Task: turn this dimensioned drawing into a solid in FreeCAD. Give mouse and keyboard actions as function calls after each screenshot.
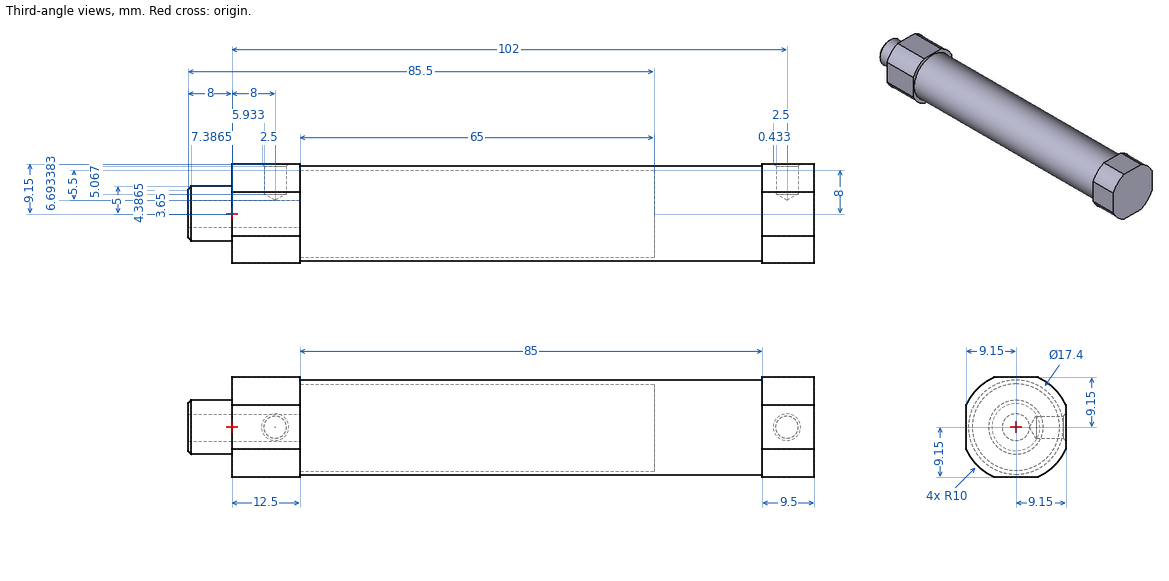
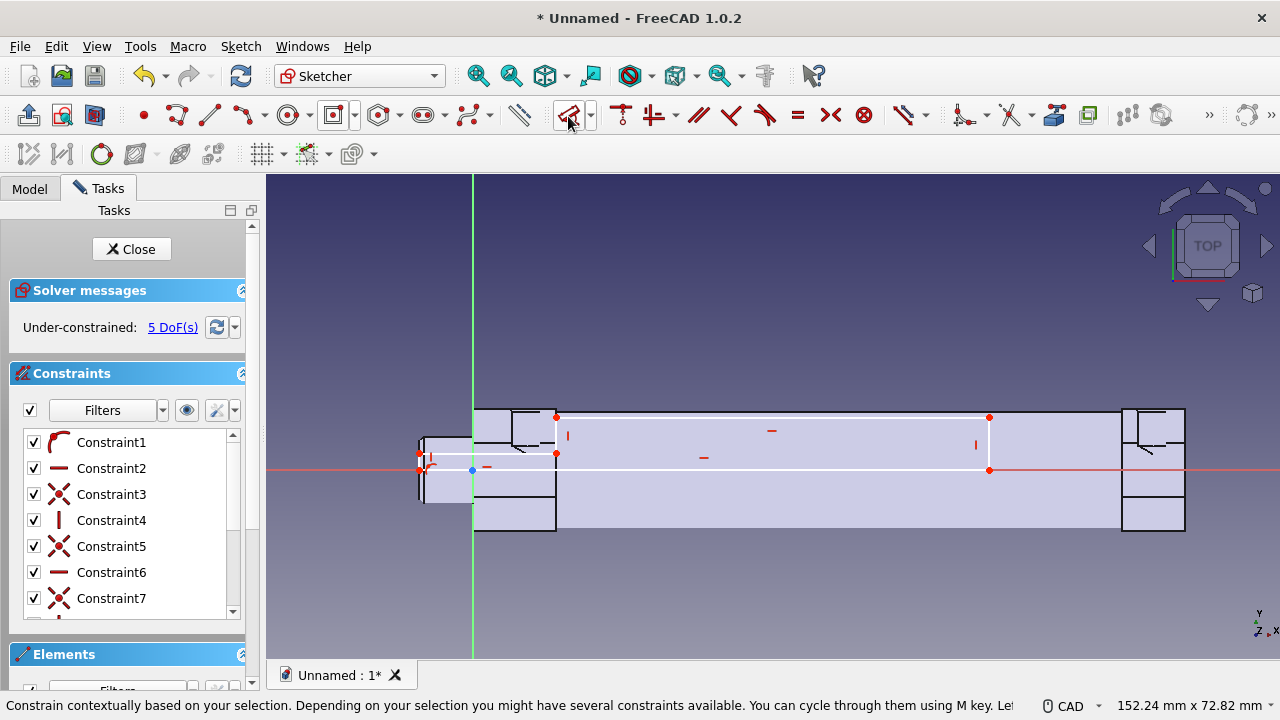
click(989, 454)
click(1023, 444)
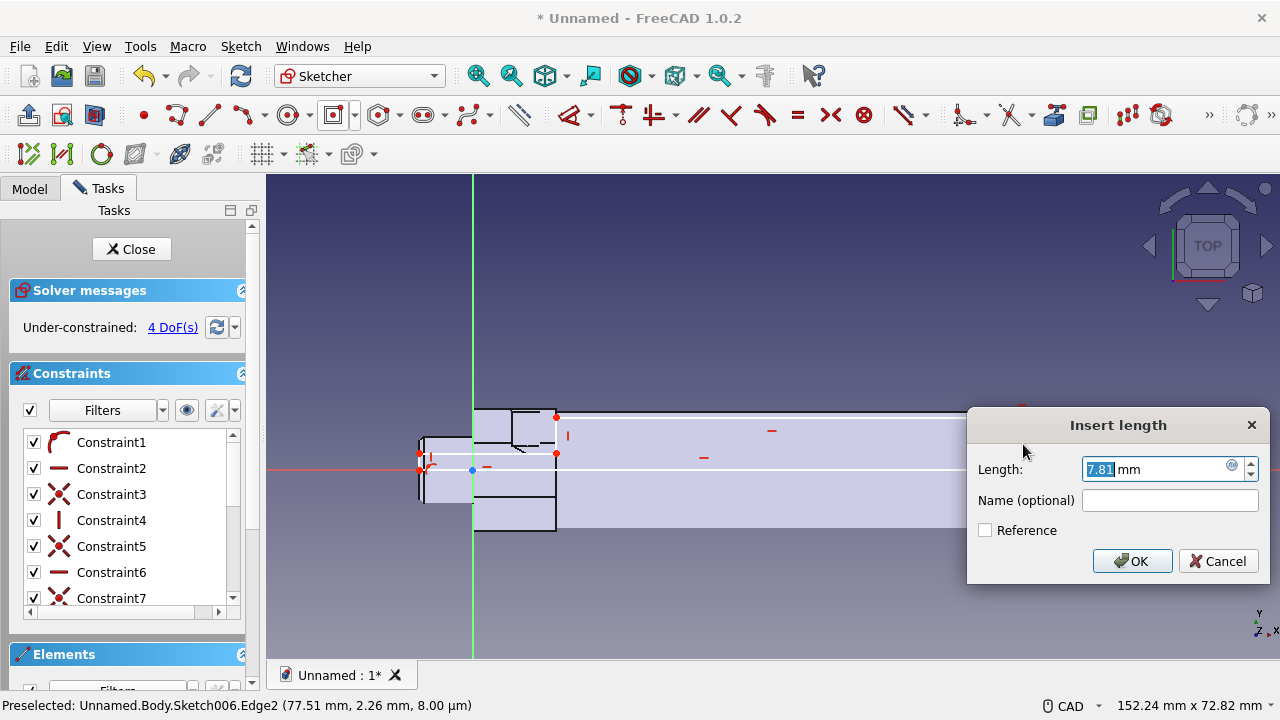
text(8)
key(Return)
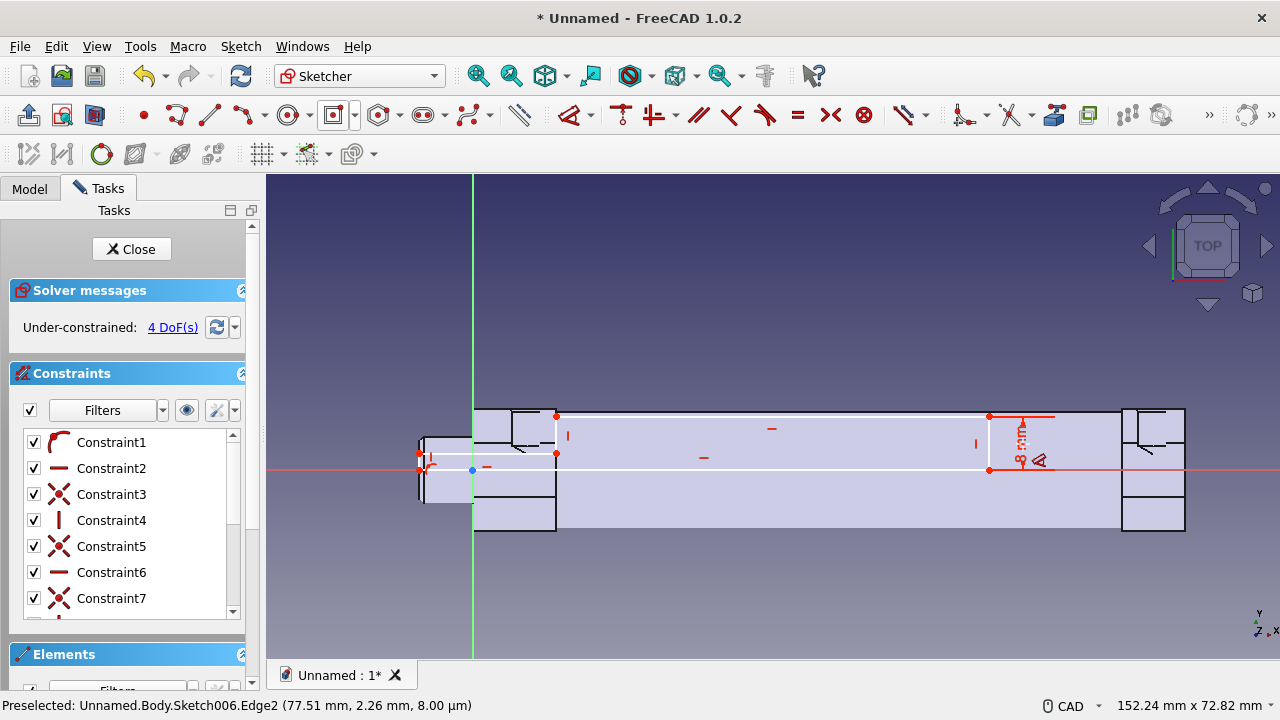
click(859, 417)
click(772, 383)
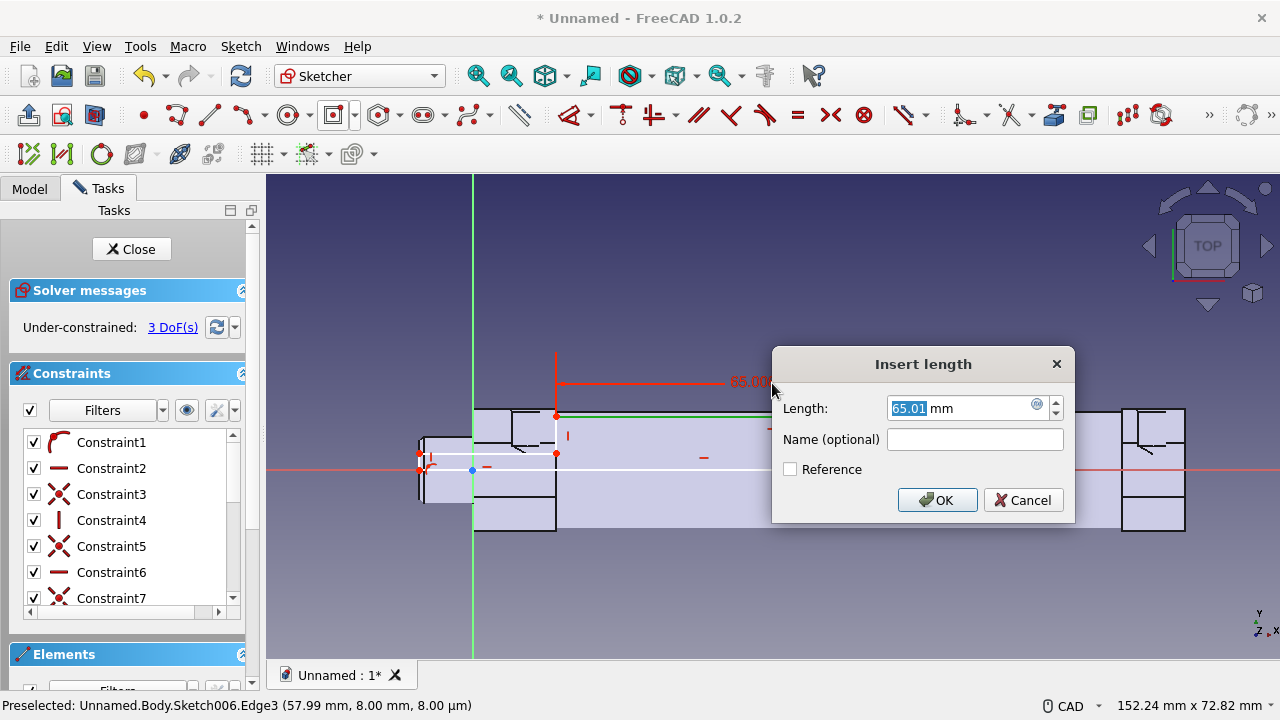
text(65)
key(Return)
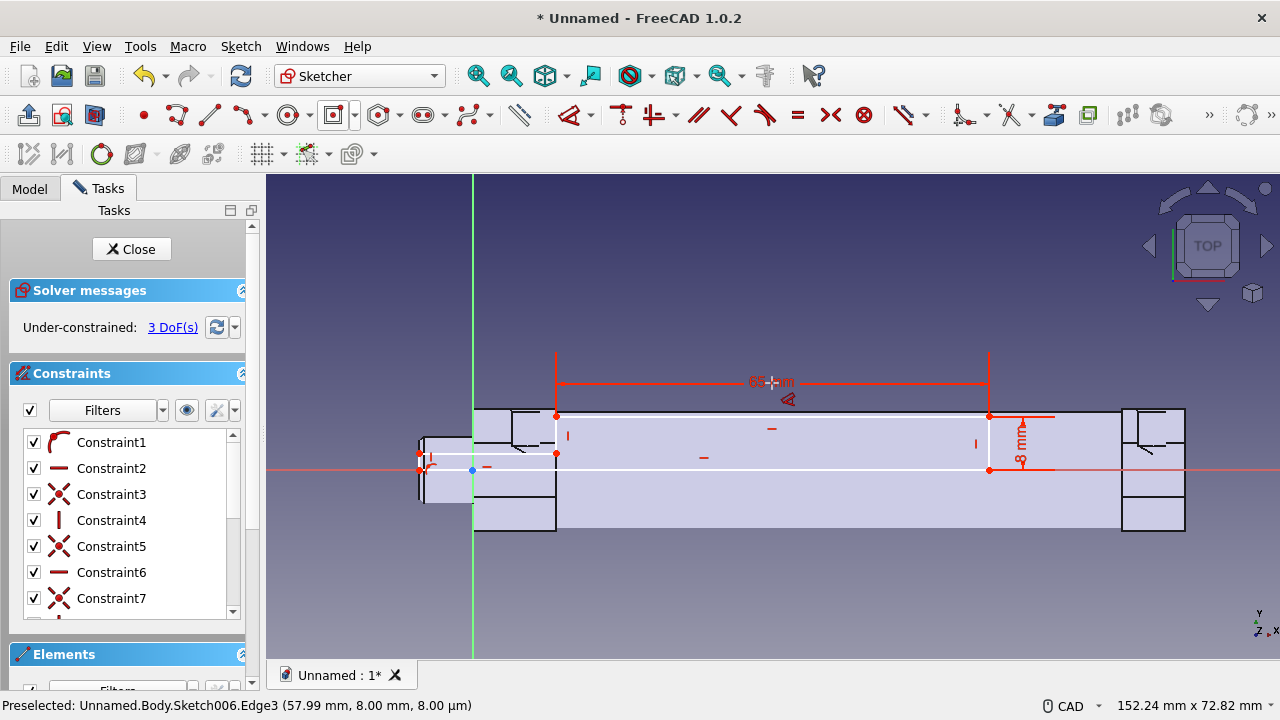
click(419, 470)
click(446, 504)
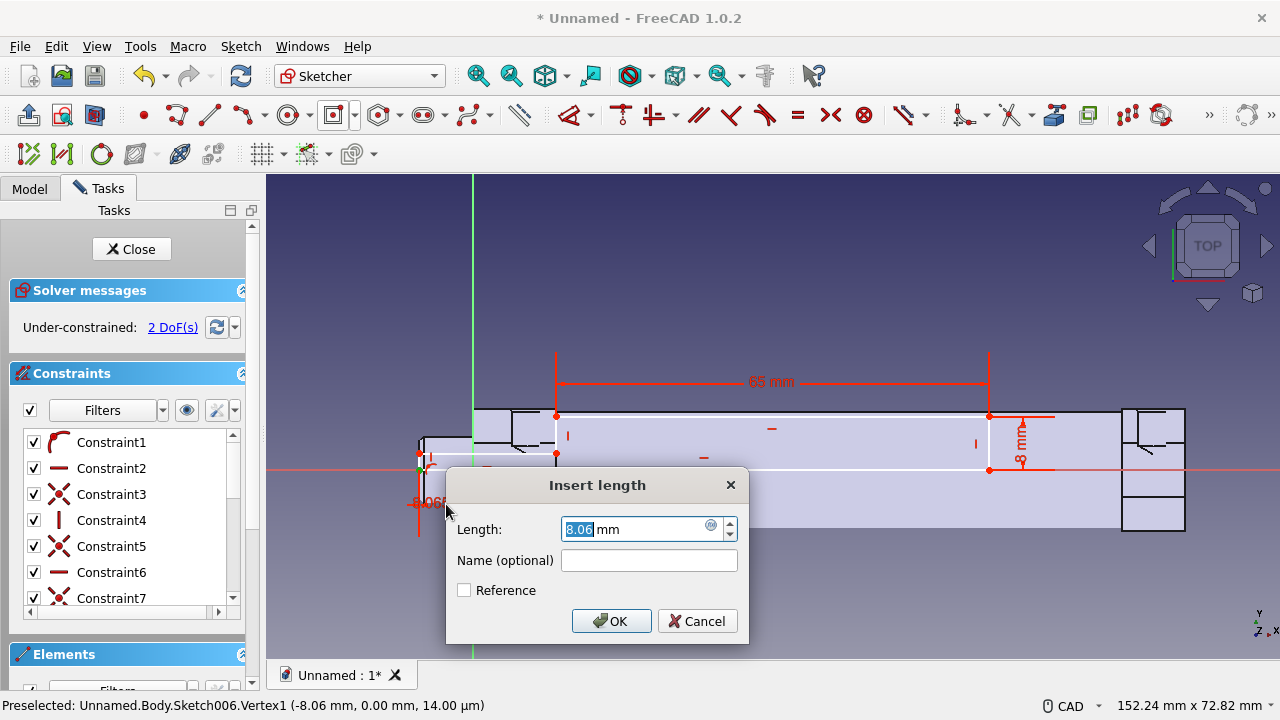
text(8)
key(Return)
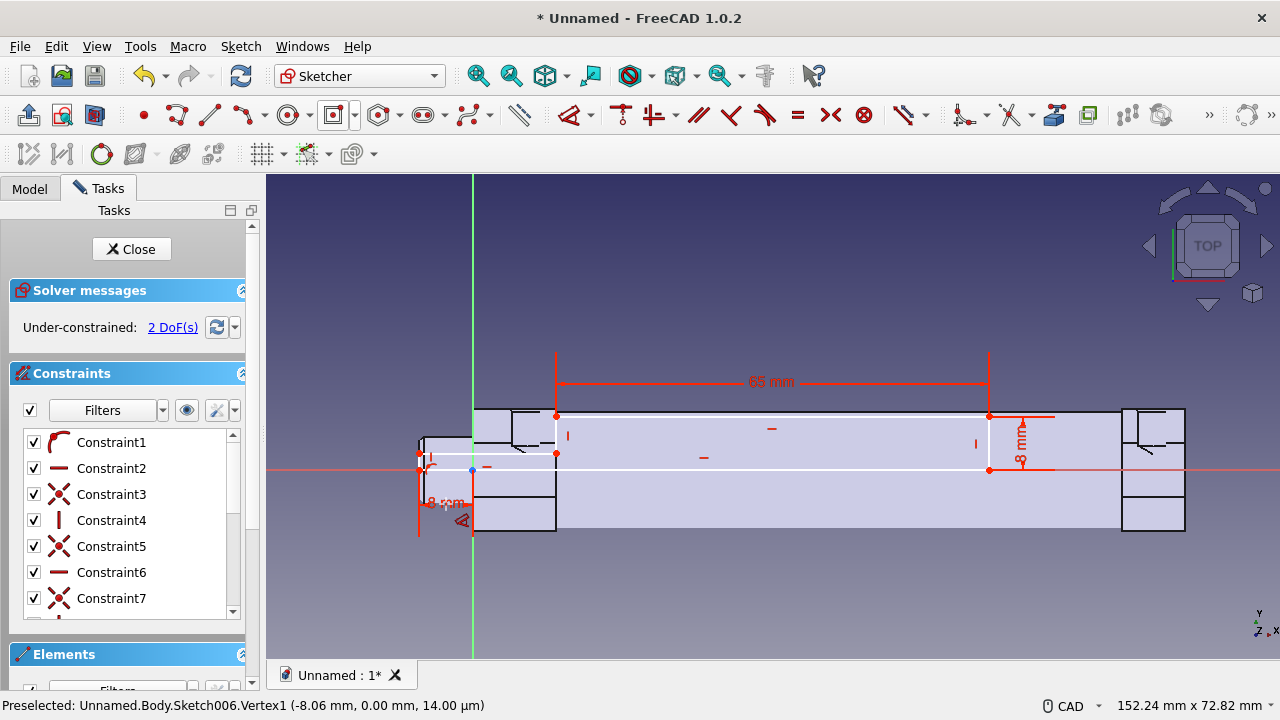
scroll(556, 428, up, 2)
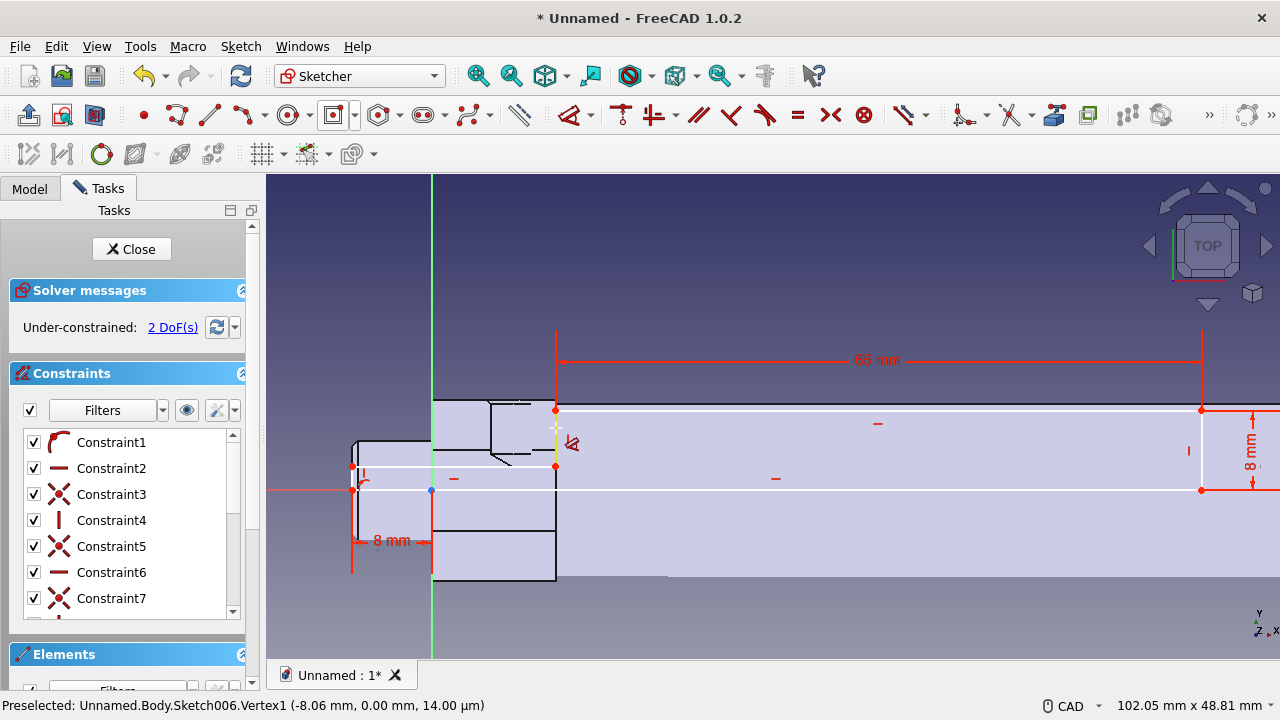
click(556, 428)
click(522, 439)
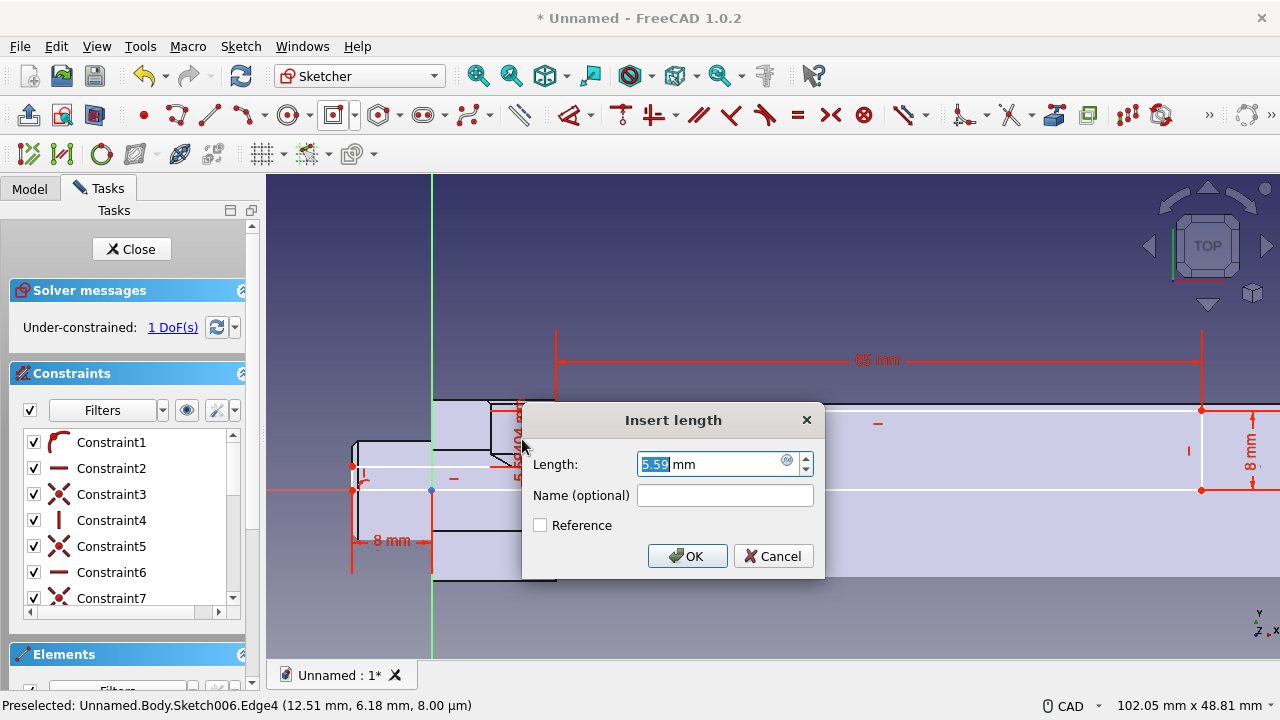
text(5.5)
key(Return)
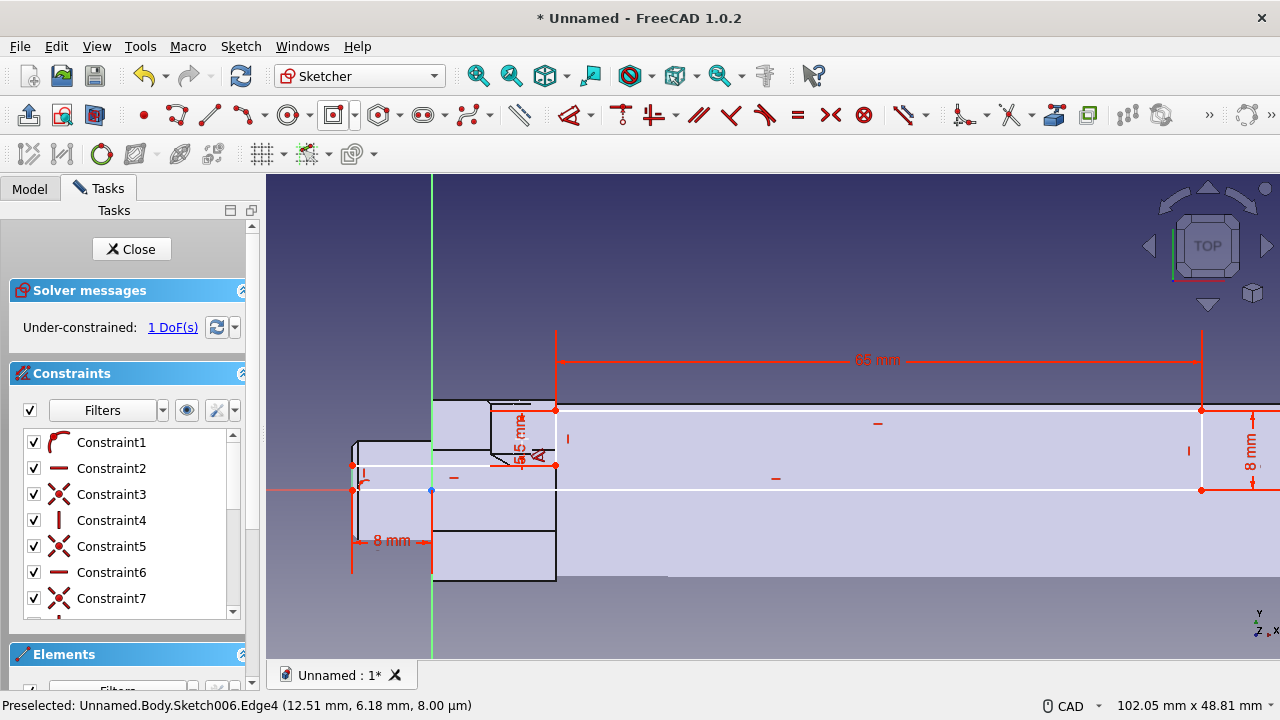
click(607, 490)
click(734, 524)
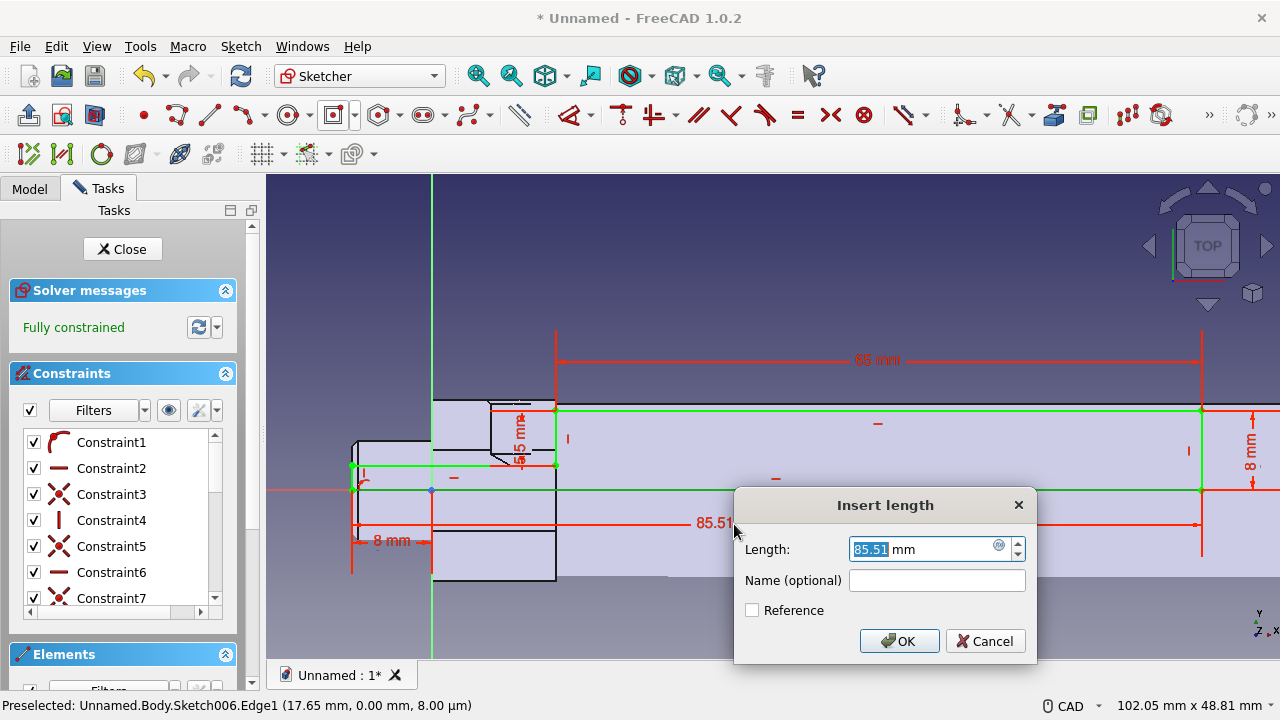
text(85.5)
key(Return)
key(Escape)